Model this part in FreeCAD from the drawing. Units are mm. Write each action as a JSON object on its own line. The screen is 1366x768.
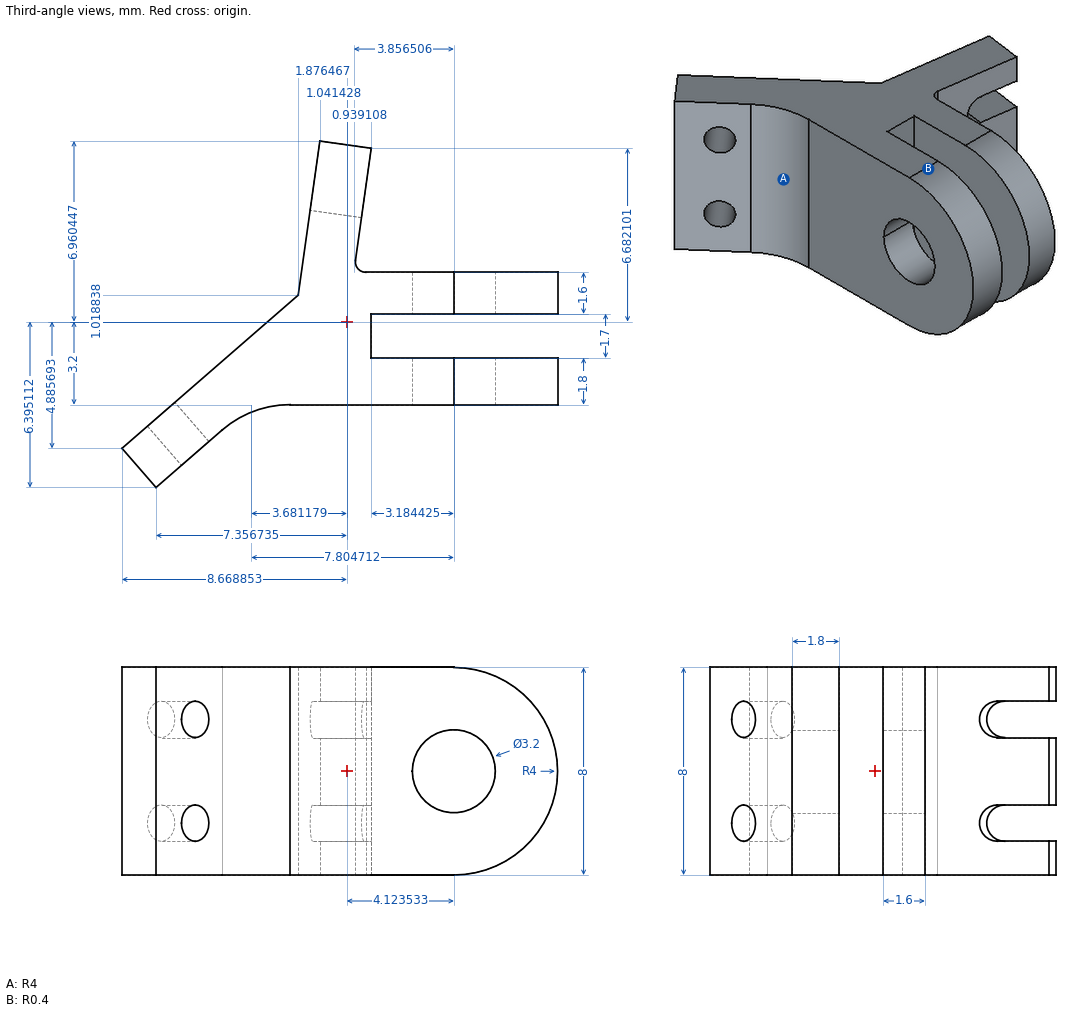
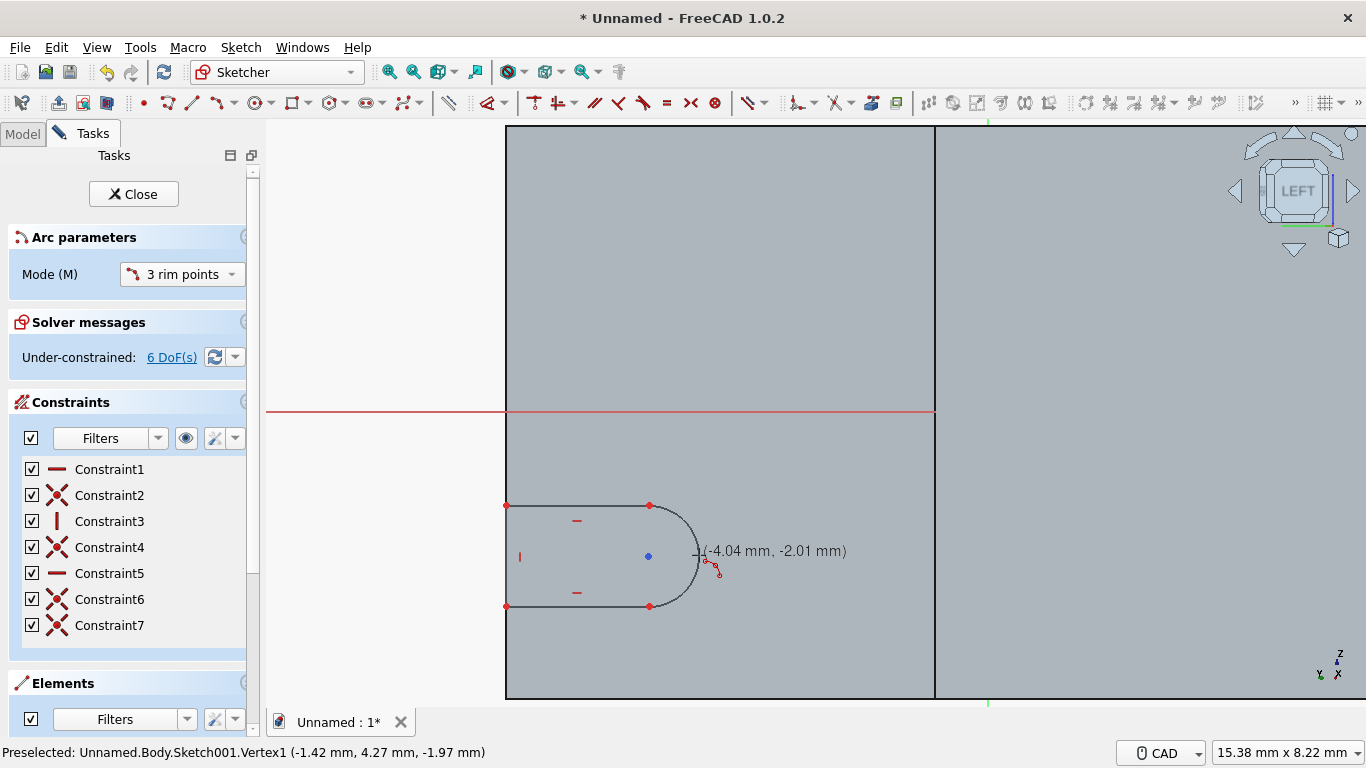
{"action": "left_click", "coordinate": [168, 104]}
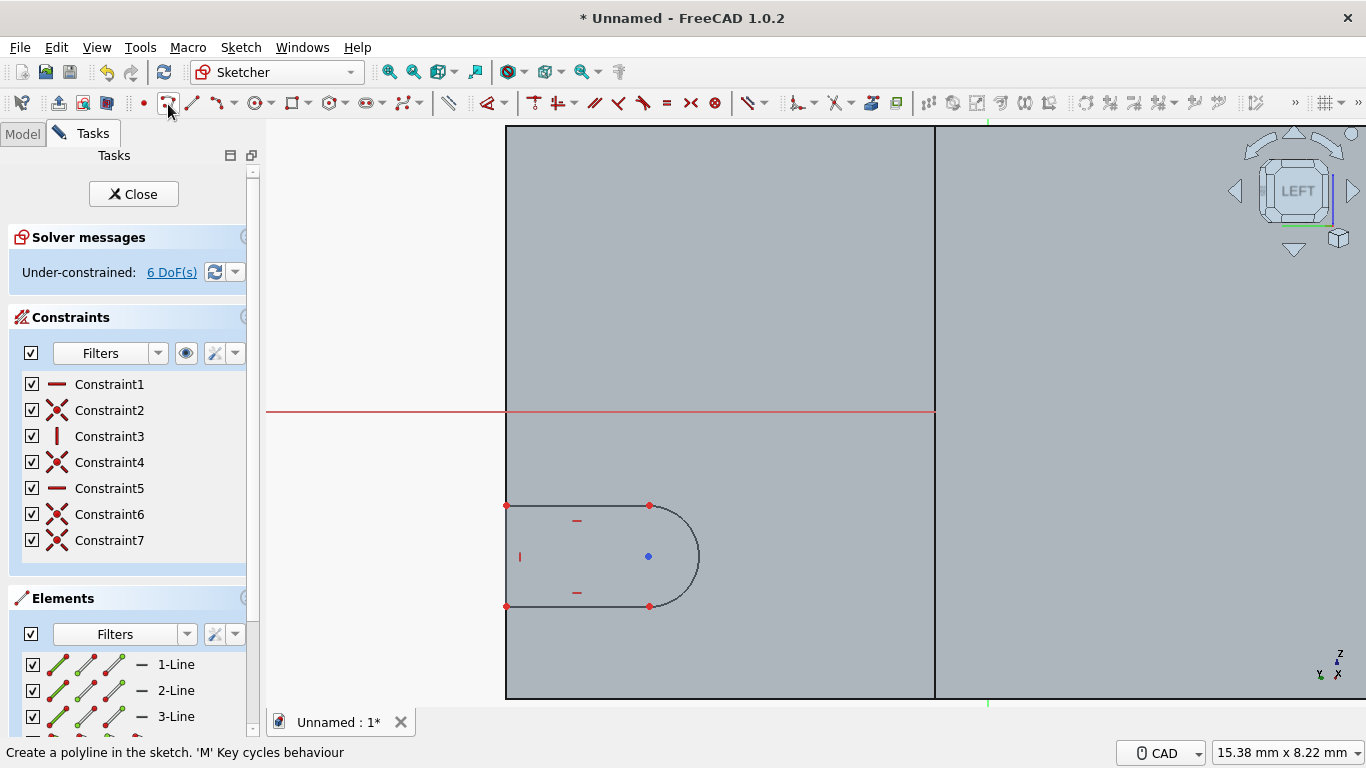
{"action": "left_click", "coordinate": [649, 219]}
{"action": "left_click", "coordinate": [506, 219]}
{"action": "left_click", "coordinate": [506, 319]}
{"action": "left_click", "coordinate": [649, 319]}
{"action": "right_click", "coordinate": [649, 319]}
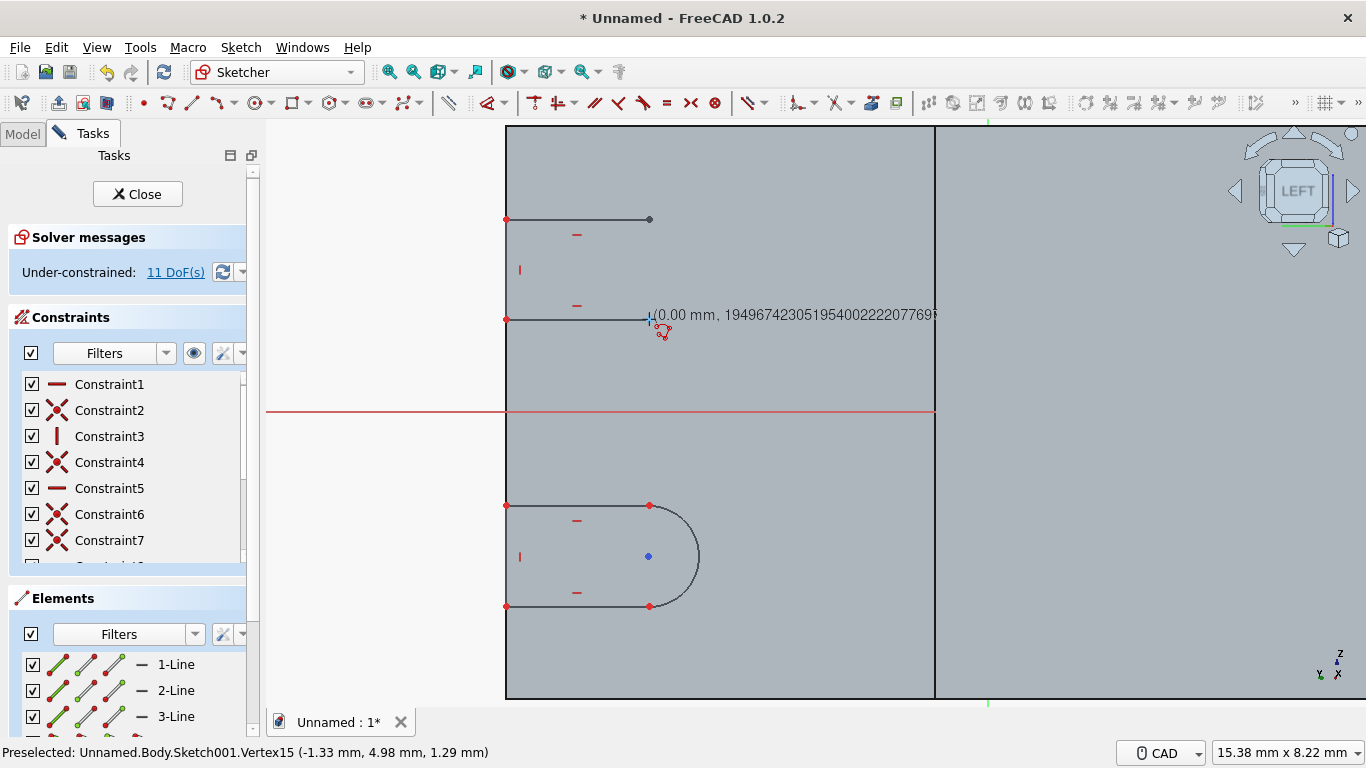
{"action": "left_click", "coordinate": [218, 104]}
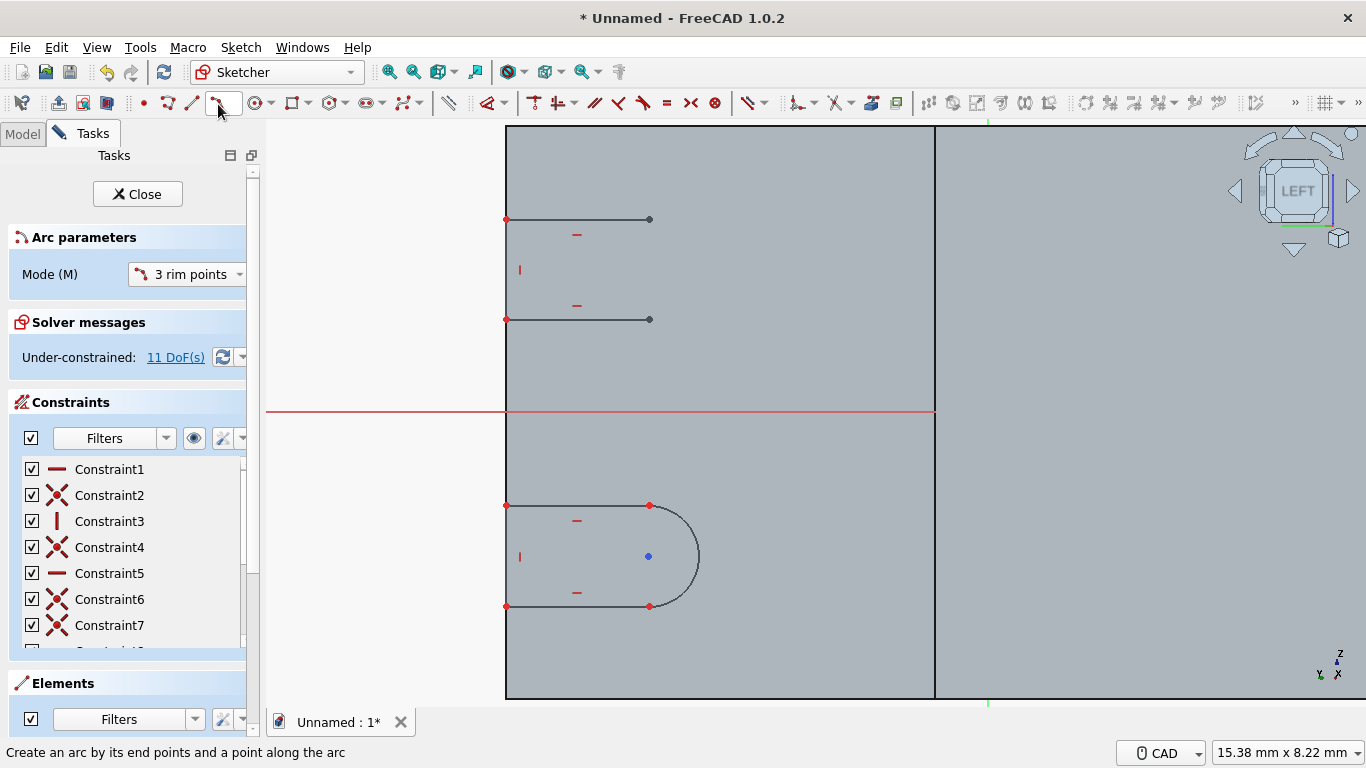
{"action": "left_click", "coordinate": [649, 320]}
{"action": "left_click", "coordinate": [649, 220]}
{"action": "left_click", "coordinate": [699, 269]}
{"action": "key", "text": "Escape"}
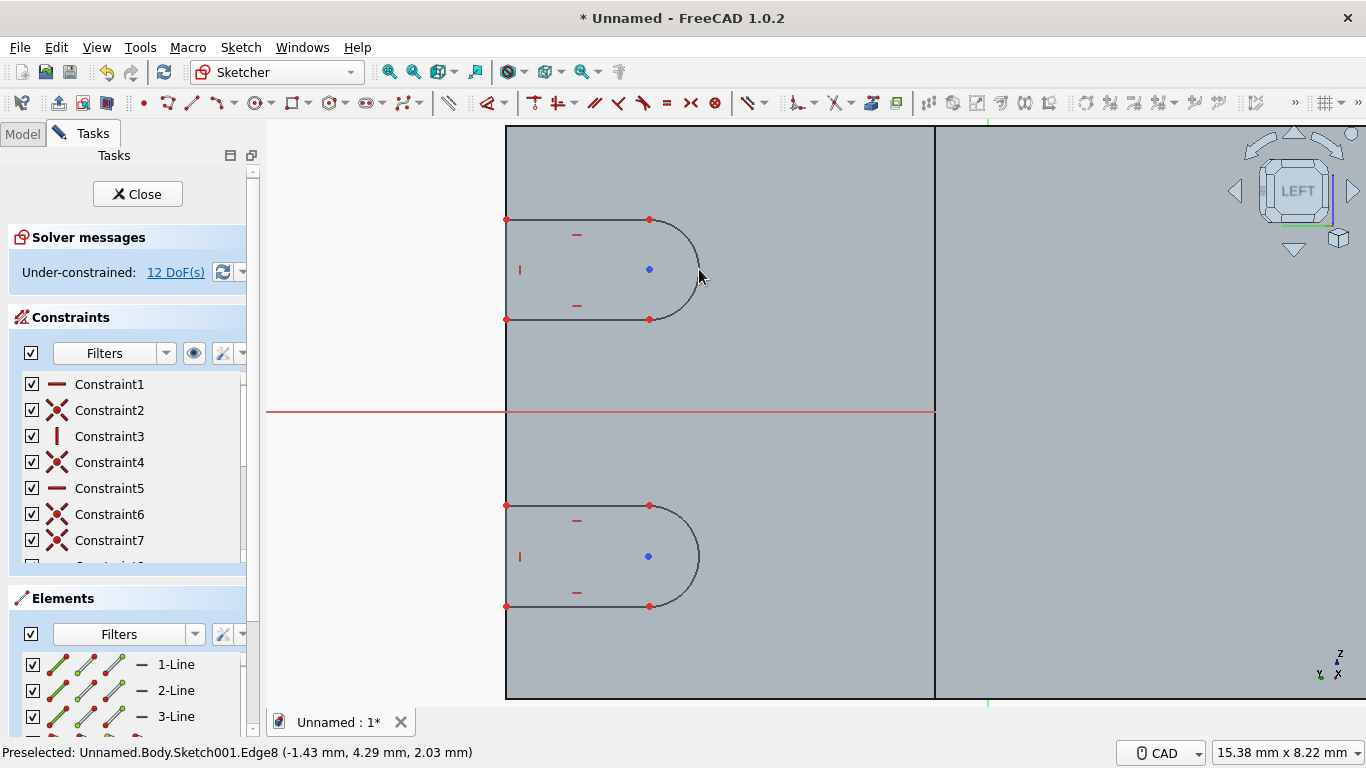
{"action": "left_click", "coordinate": [606, 506]}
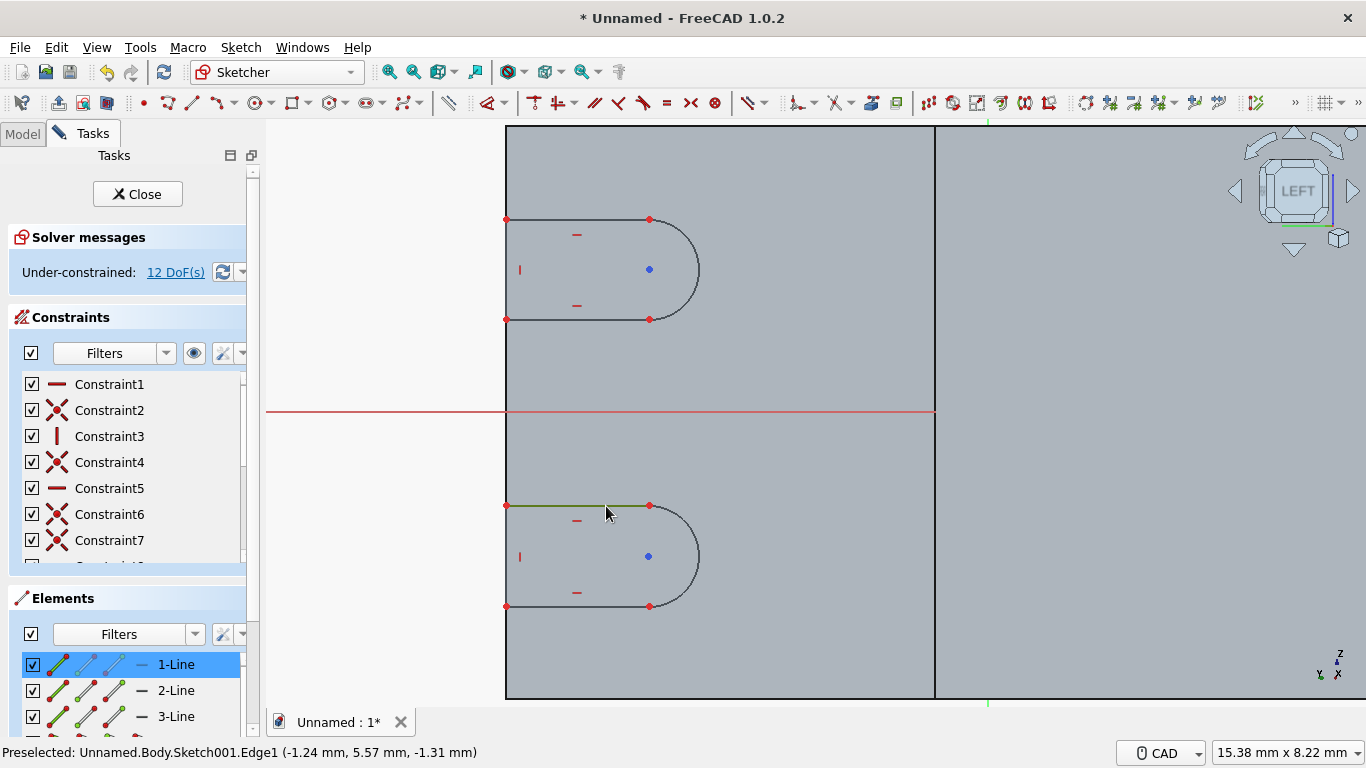
{"action": "left_click", "coordinate": [689, 586]}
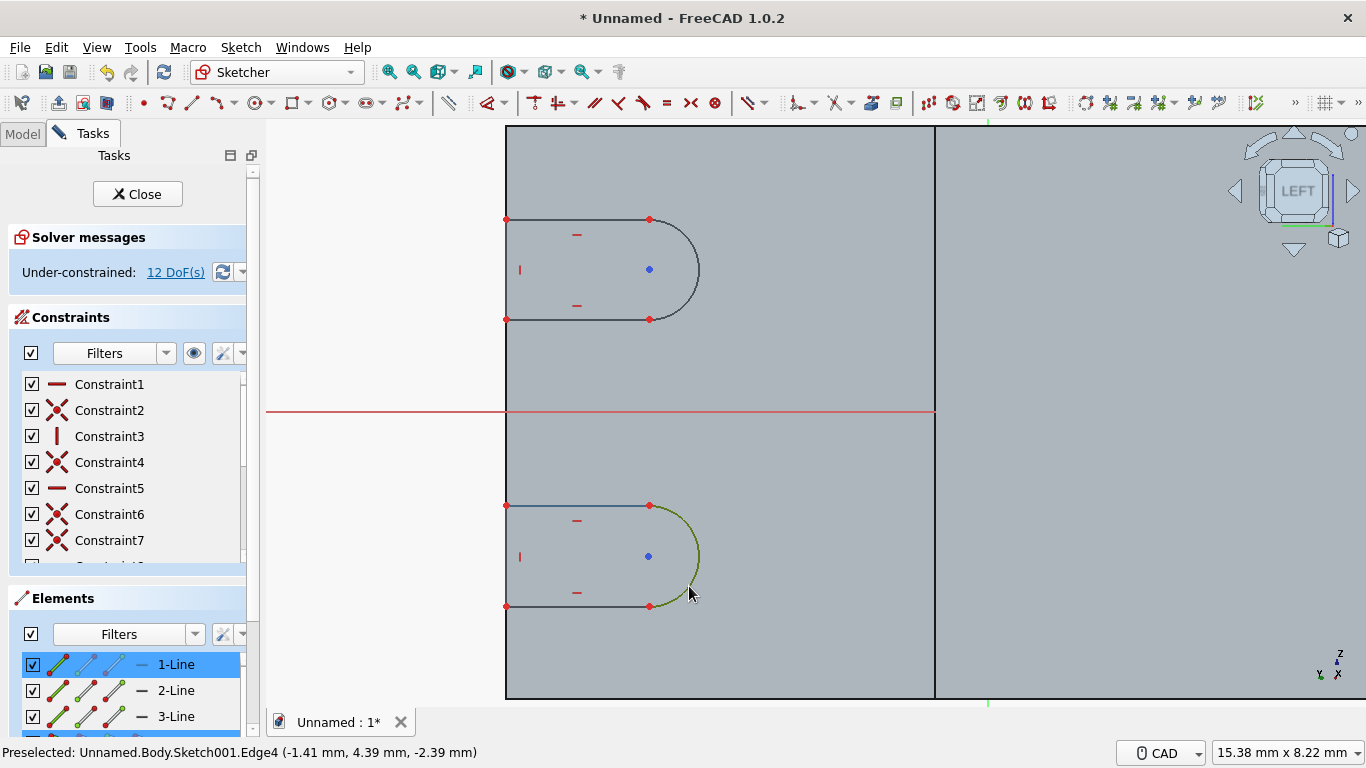
{"action": "left_click", "coordinate": [644, 104]}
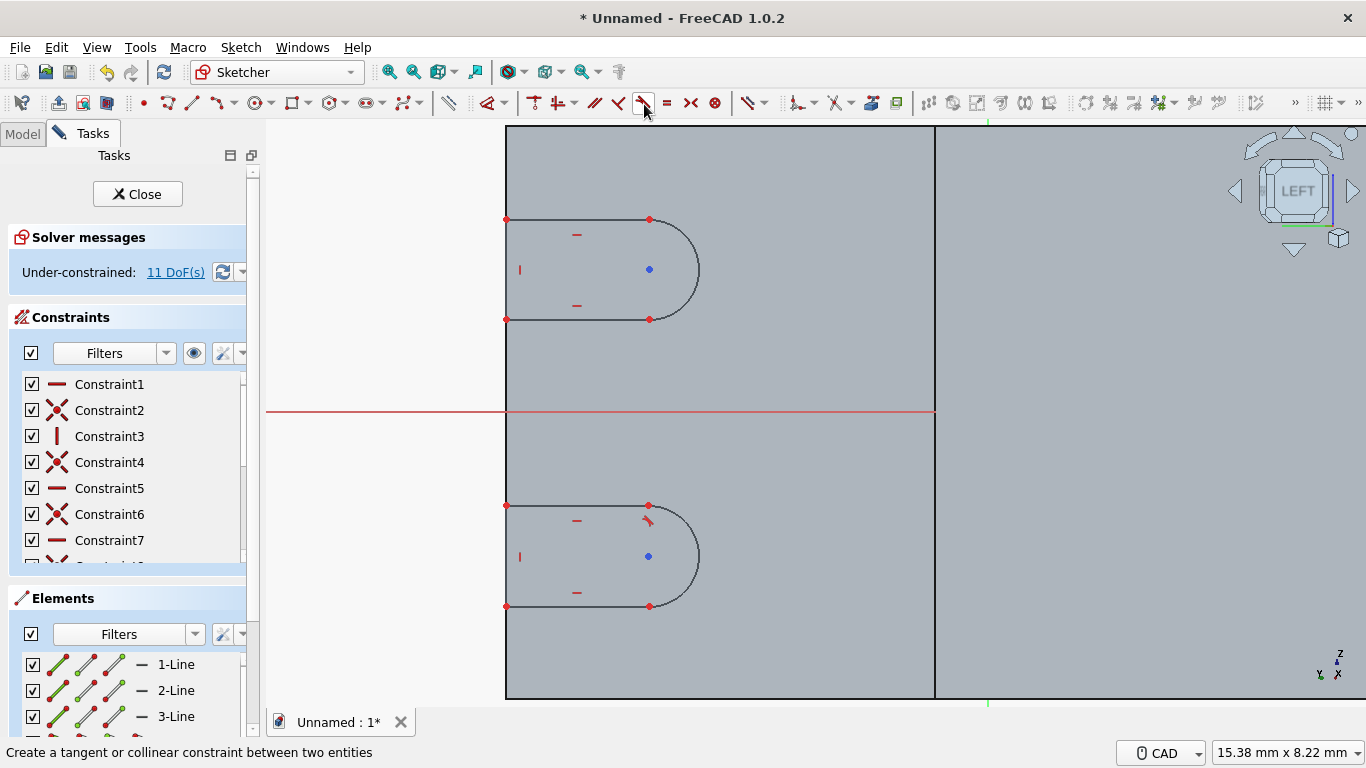
{"action": "left_click", "coordinate": [549, 607]}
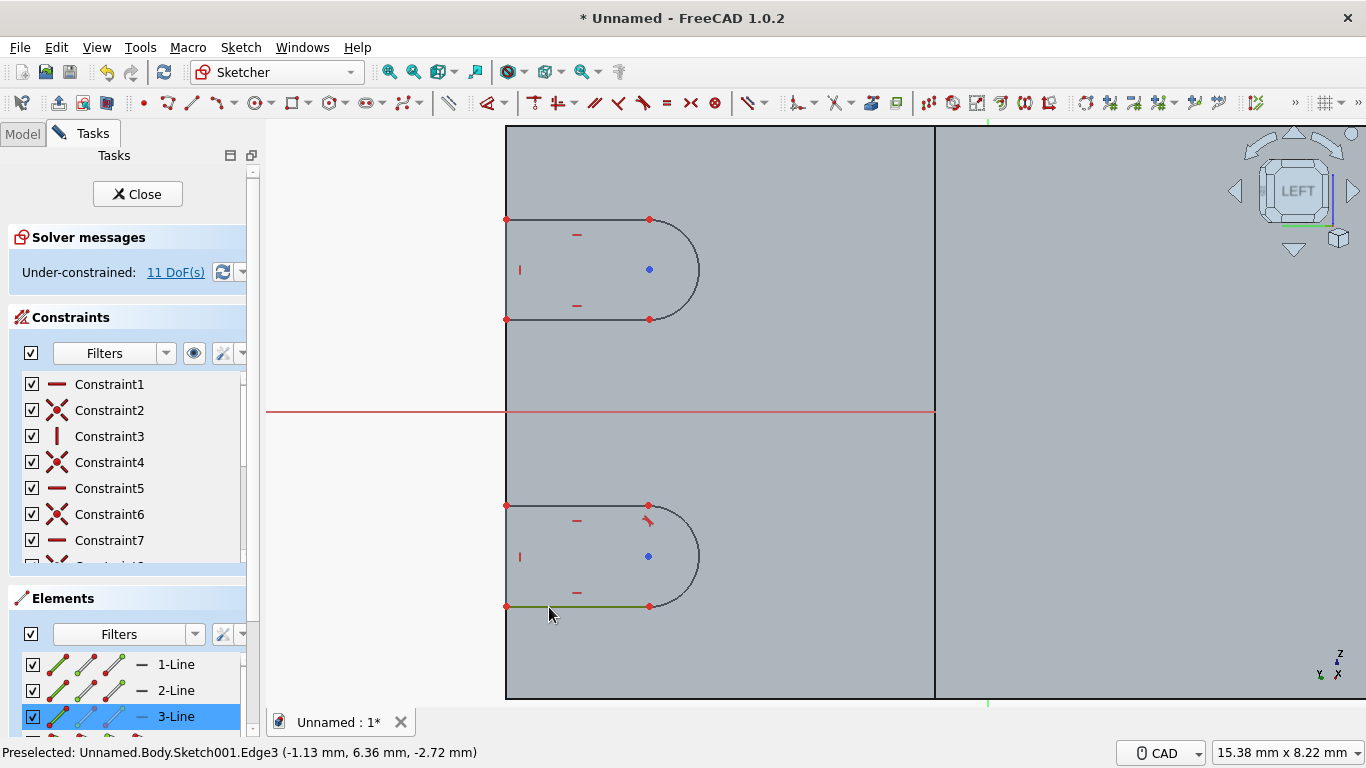
{"action": "left_click", "coordinate": [690, 586]}